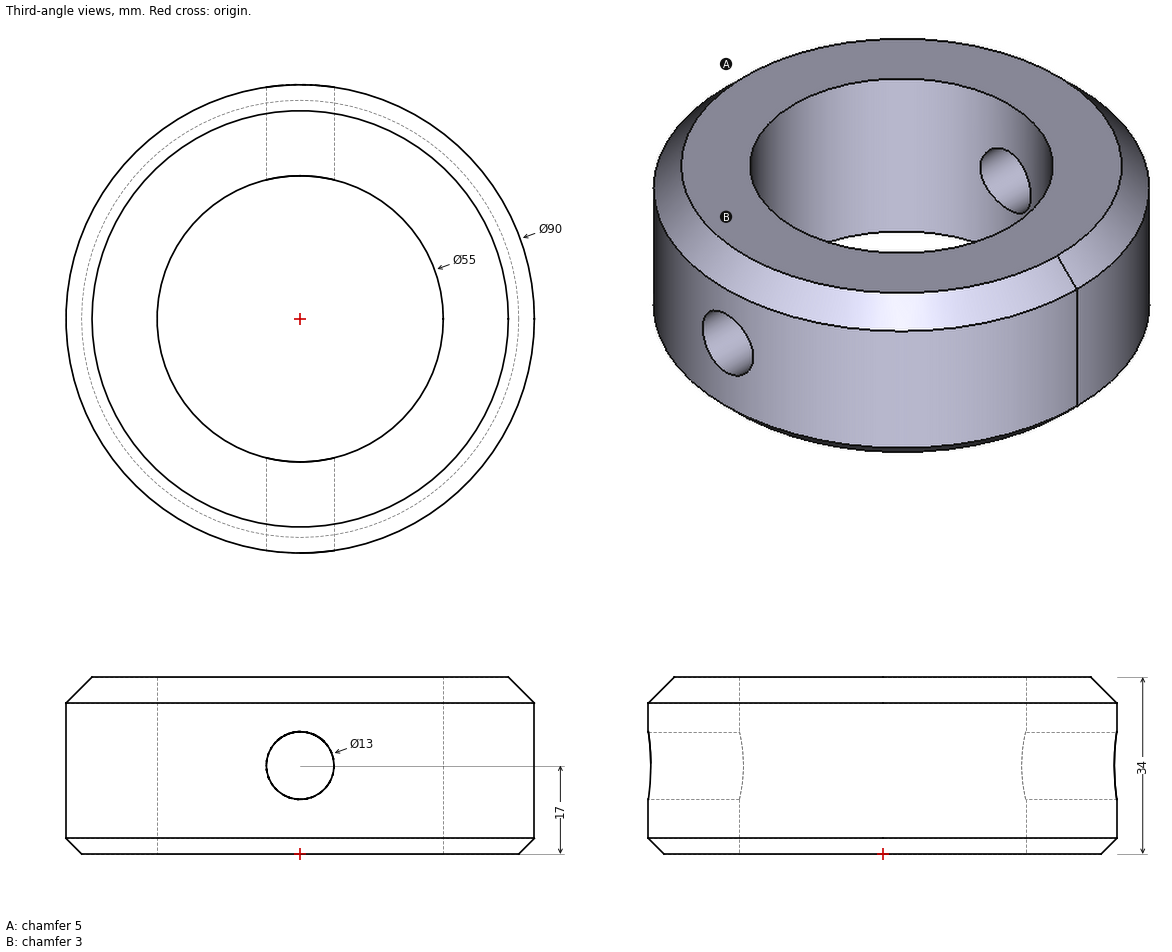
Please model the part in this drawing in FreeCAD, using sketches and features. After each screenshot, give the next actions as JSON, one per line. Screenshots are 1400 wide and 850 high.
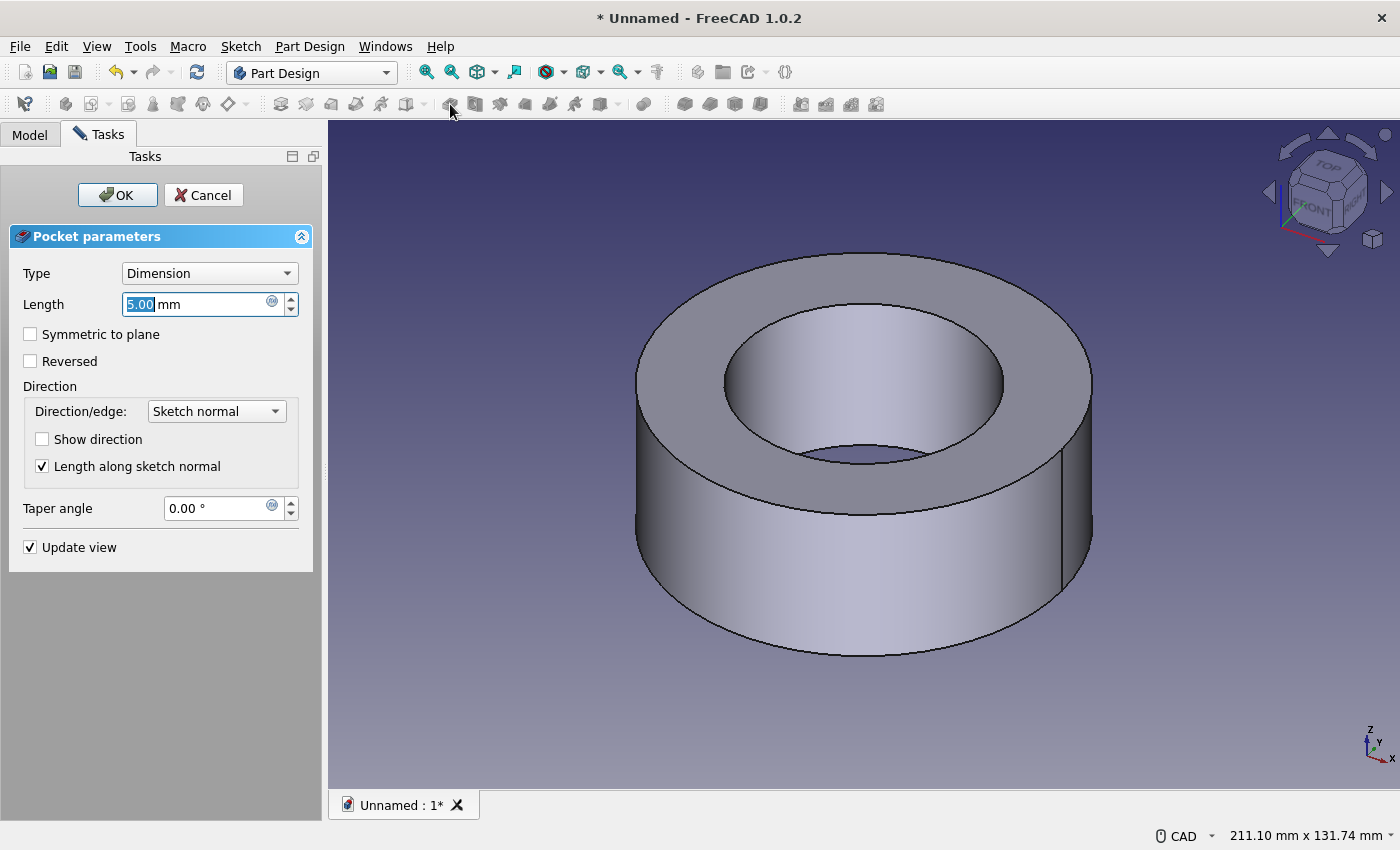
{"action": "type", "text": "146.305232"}
{"action": "key", "text": "Tab"}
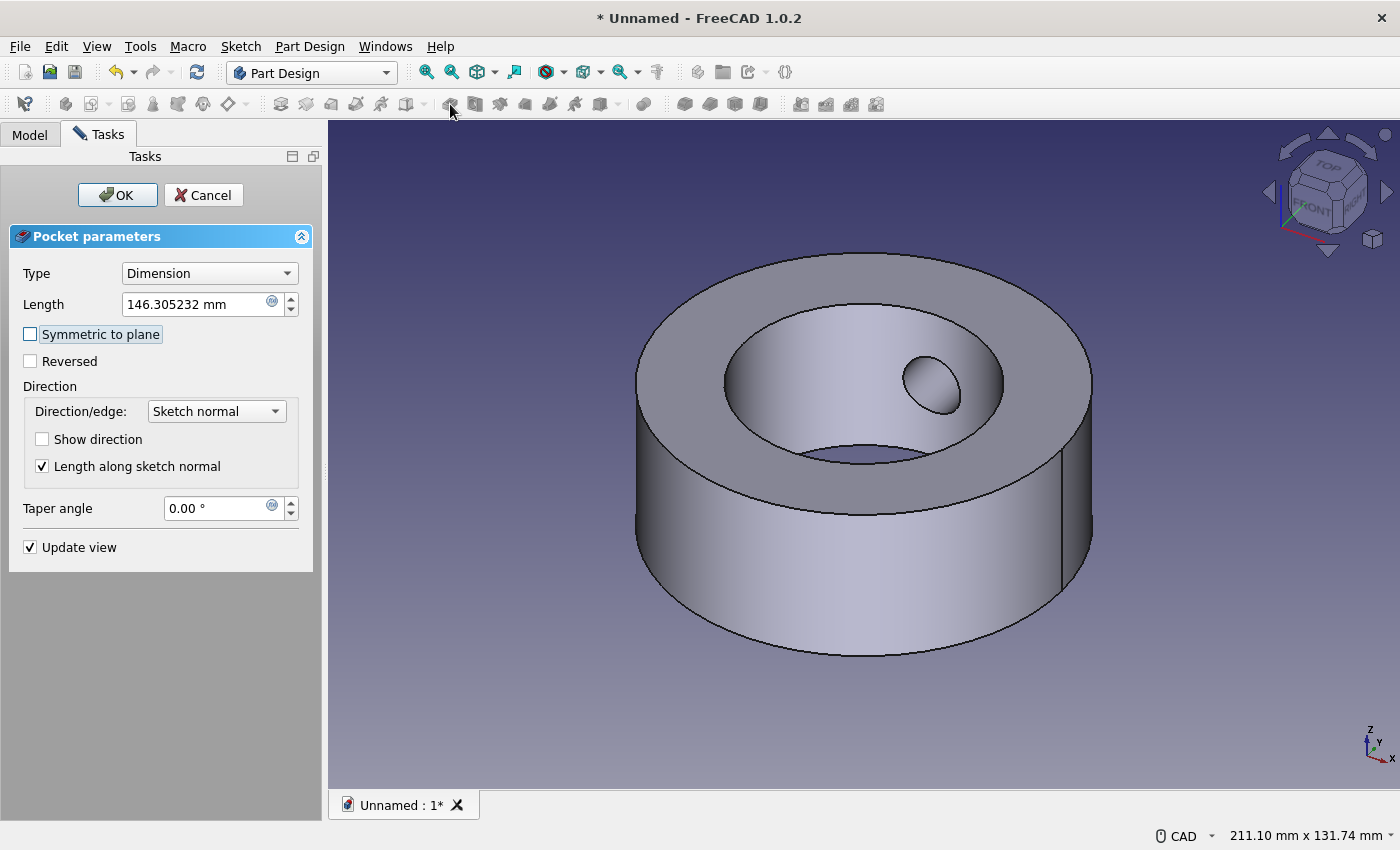
{"action": "left_click", "coordinate": [31, 334]}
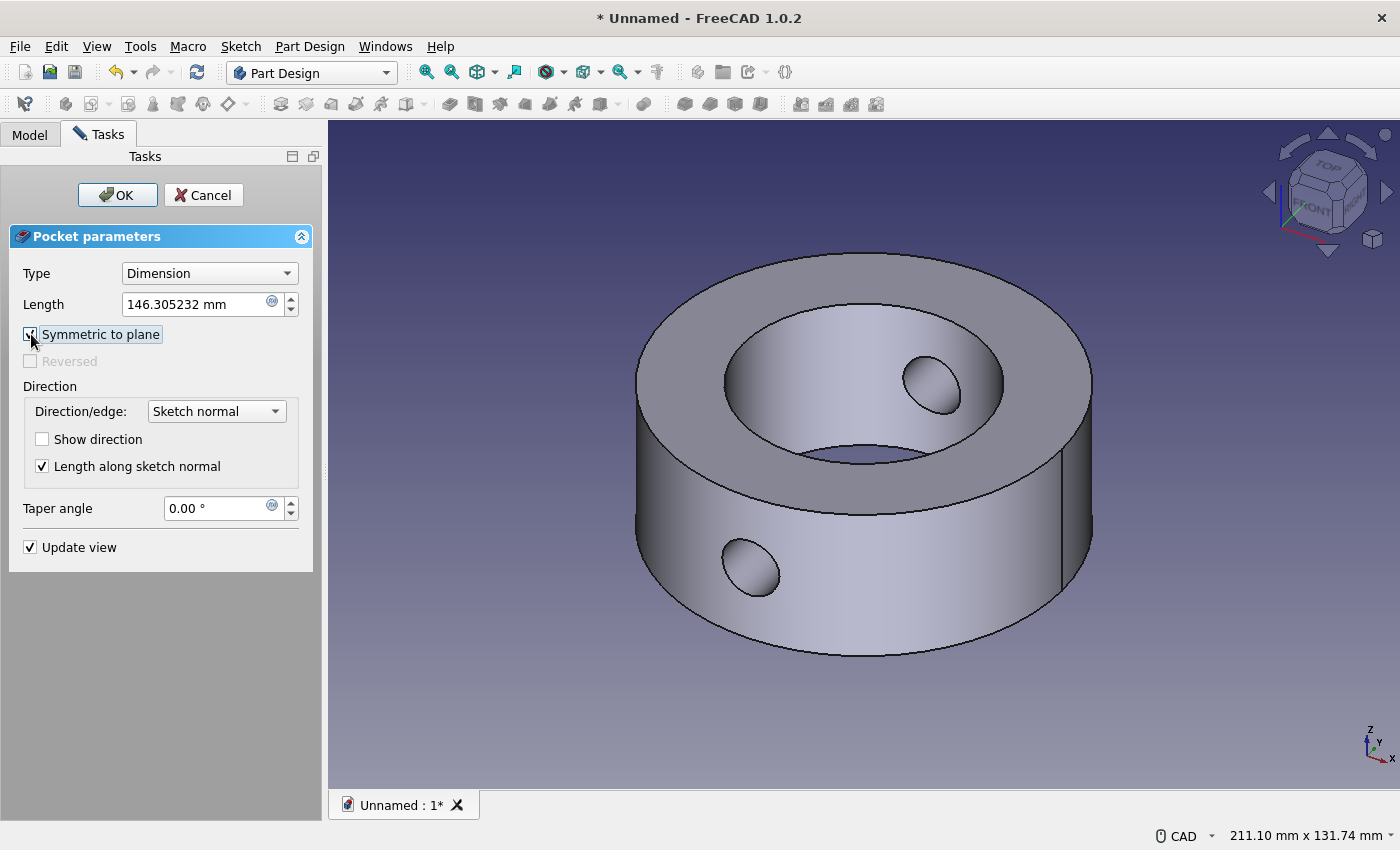
{"action": "left_click", "coordinate": [118, 195]}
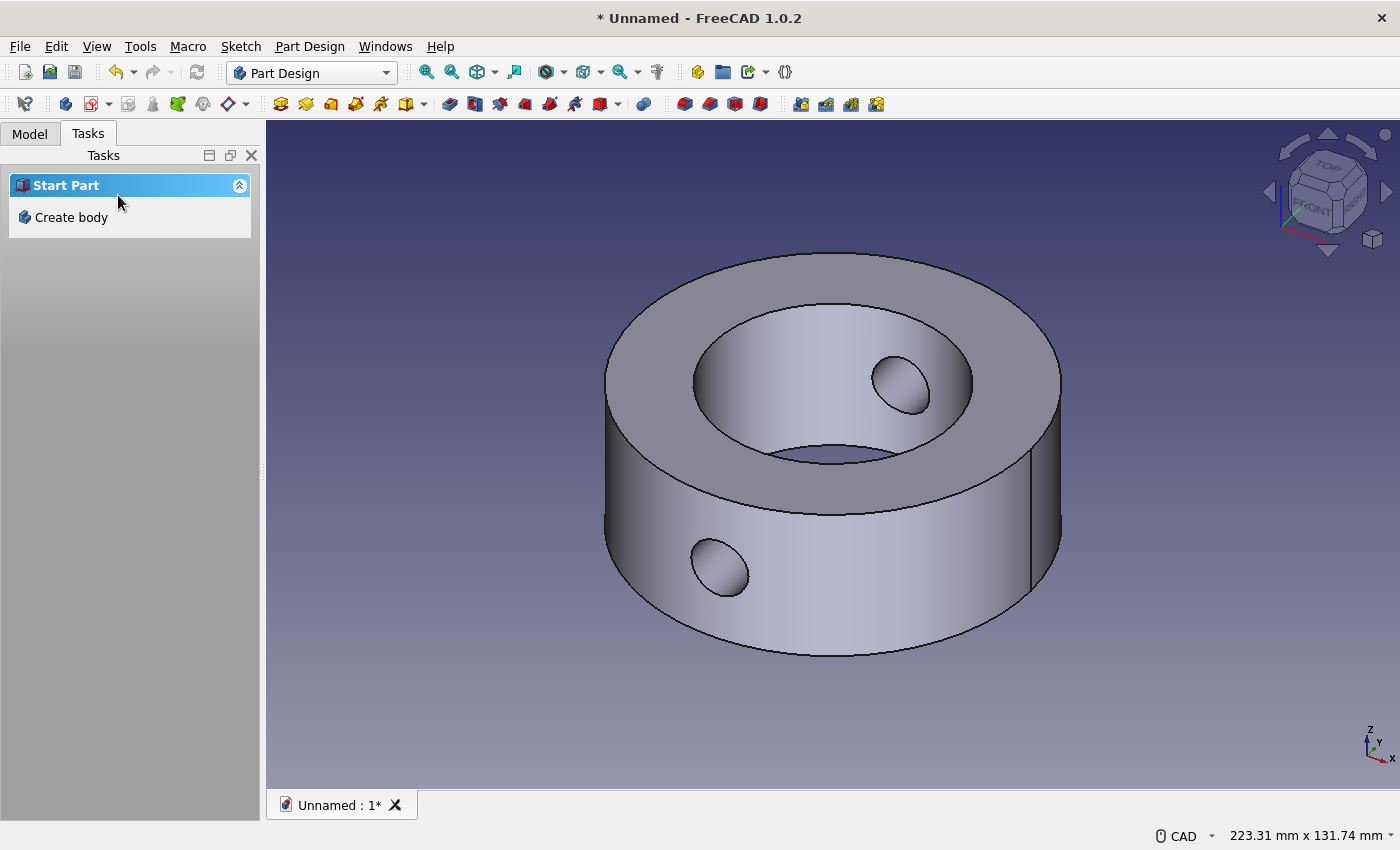
{"action": "left_click", "coordinate": [606, 396]}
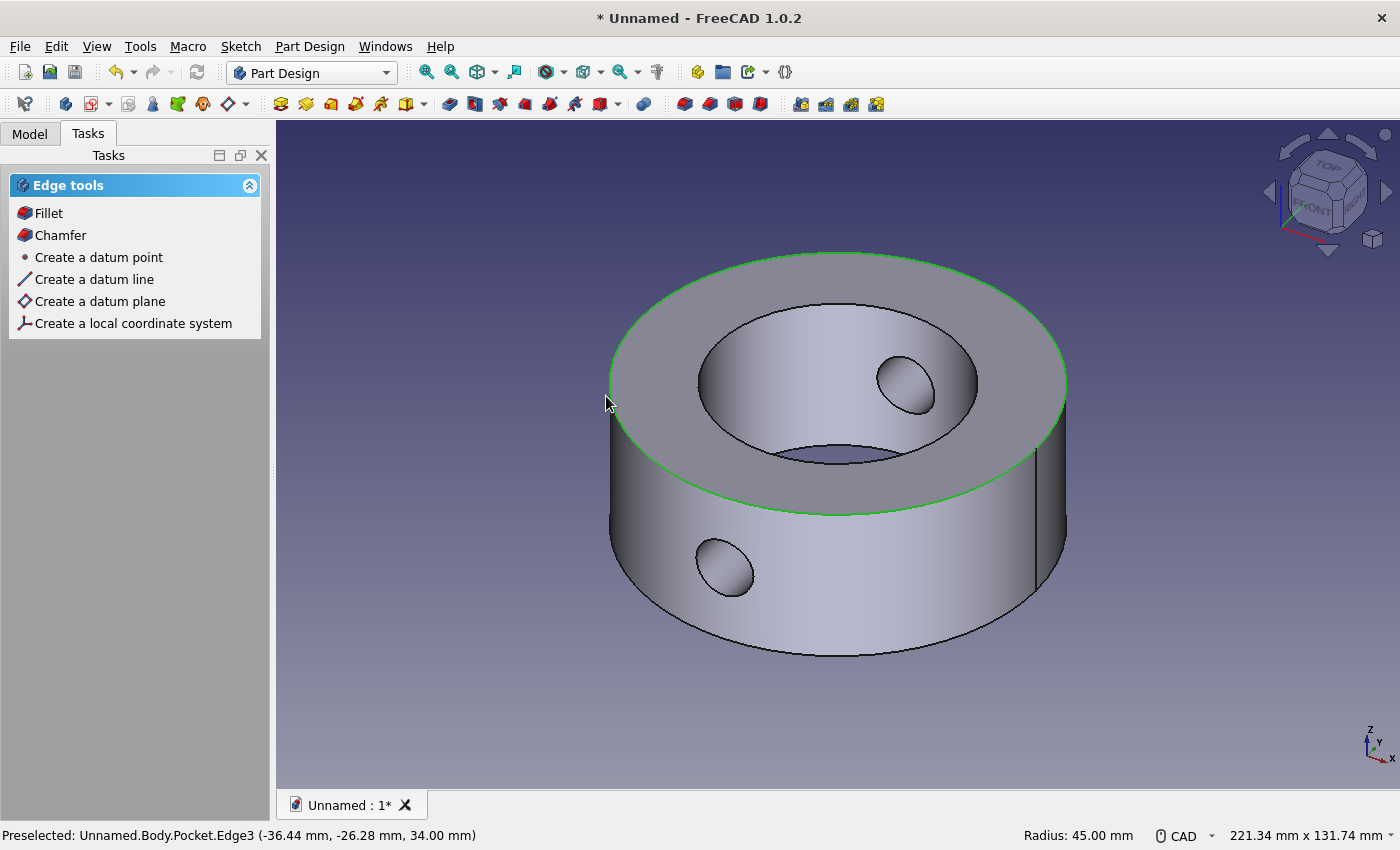
{"action": "left_click", "coordinate": [710, 104]}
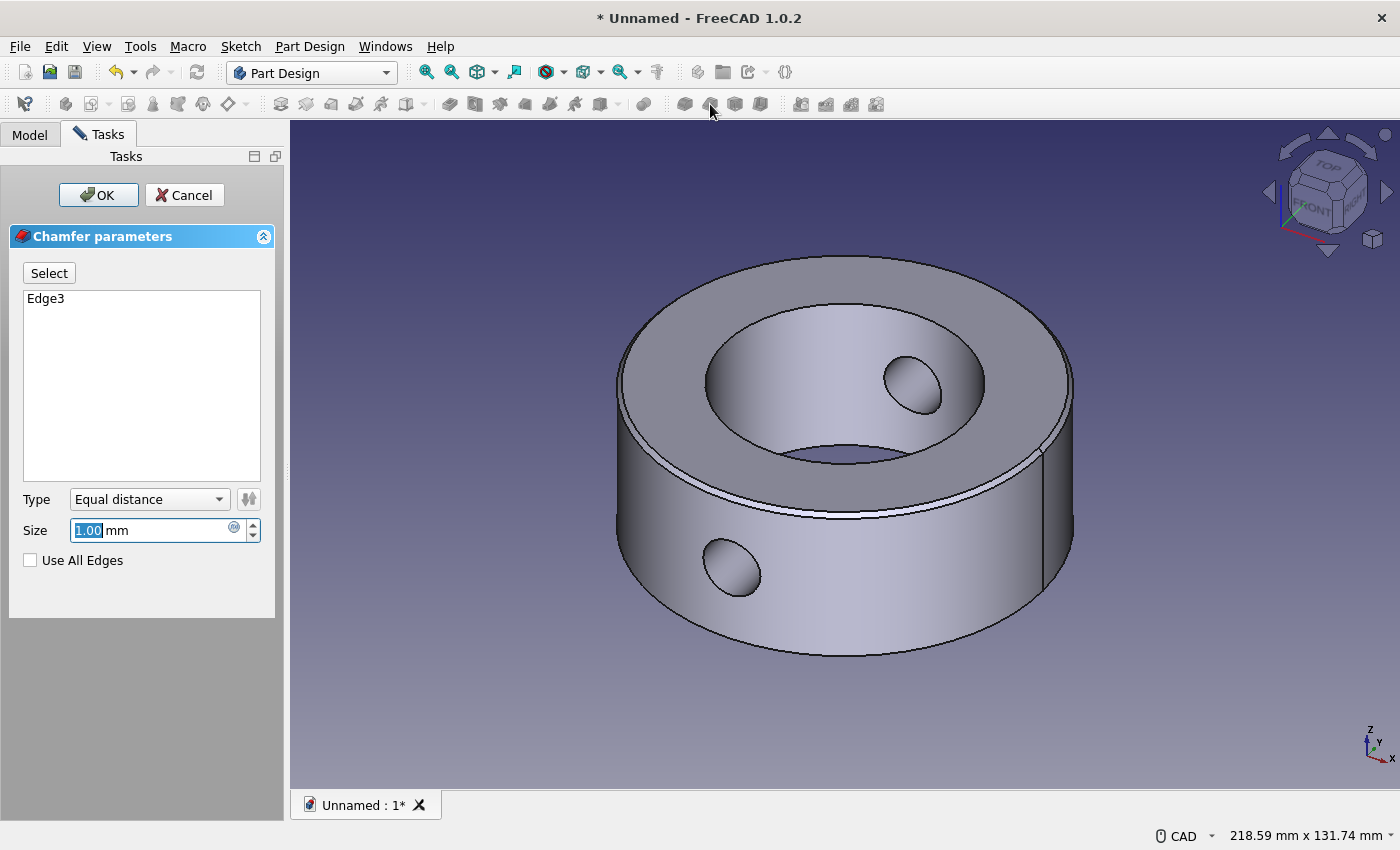
{"action": "type", "text": "5"}
{"action": "key", "text": "Tab"}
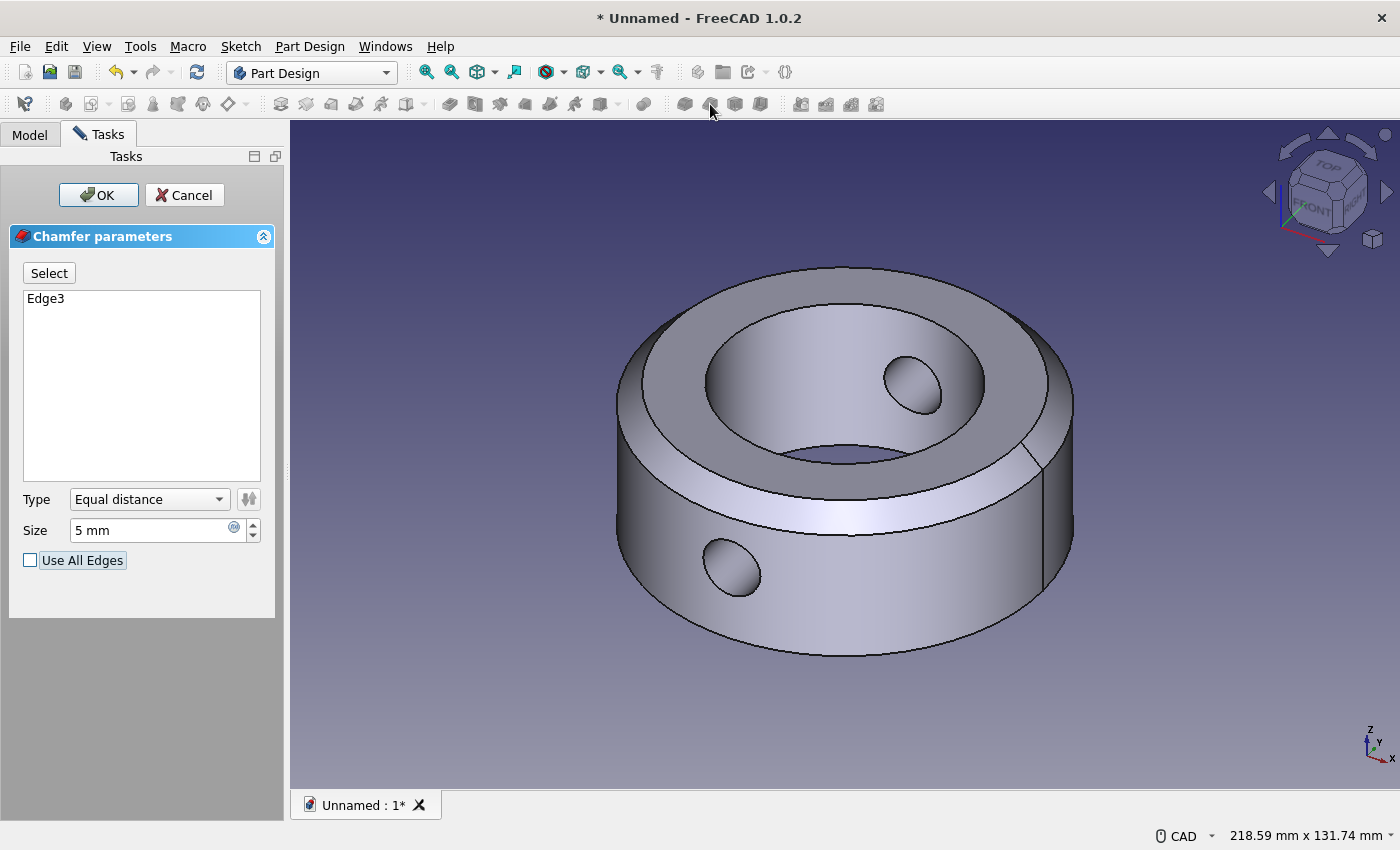
{"action": "left_click", "coordinate": [99, 195]}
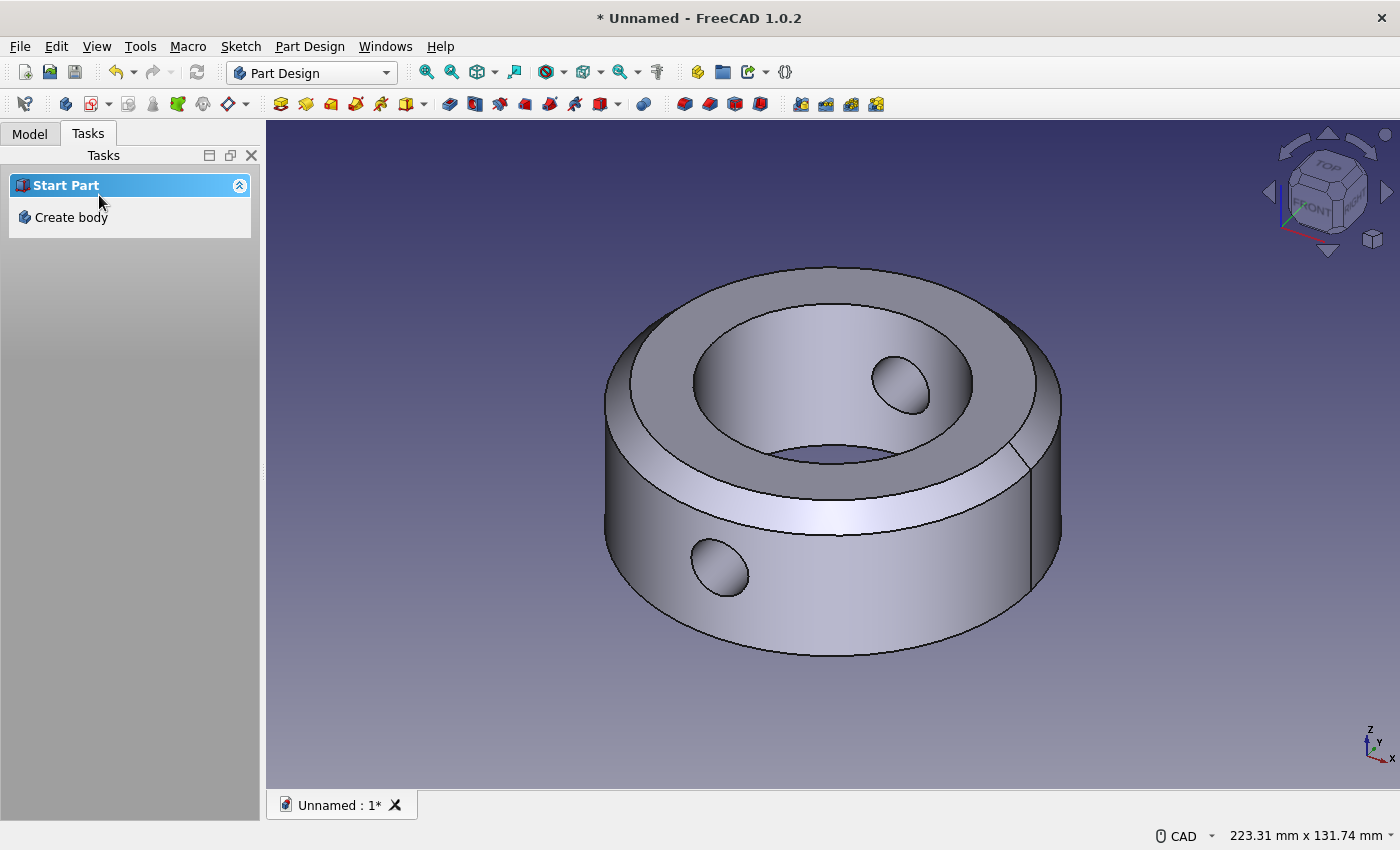
{"action": "key", "text": "0"}